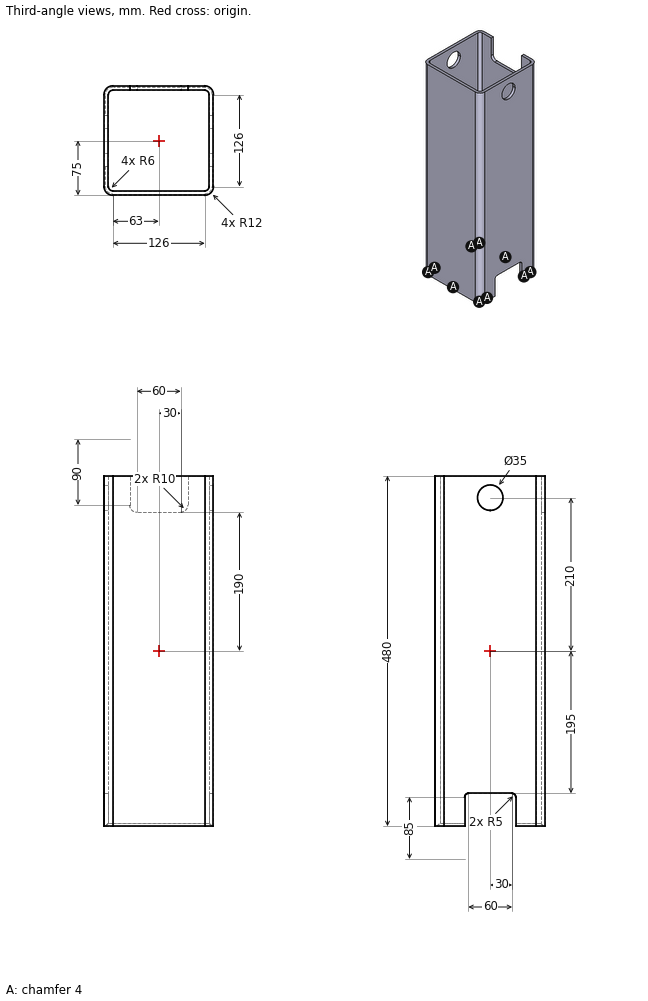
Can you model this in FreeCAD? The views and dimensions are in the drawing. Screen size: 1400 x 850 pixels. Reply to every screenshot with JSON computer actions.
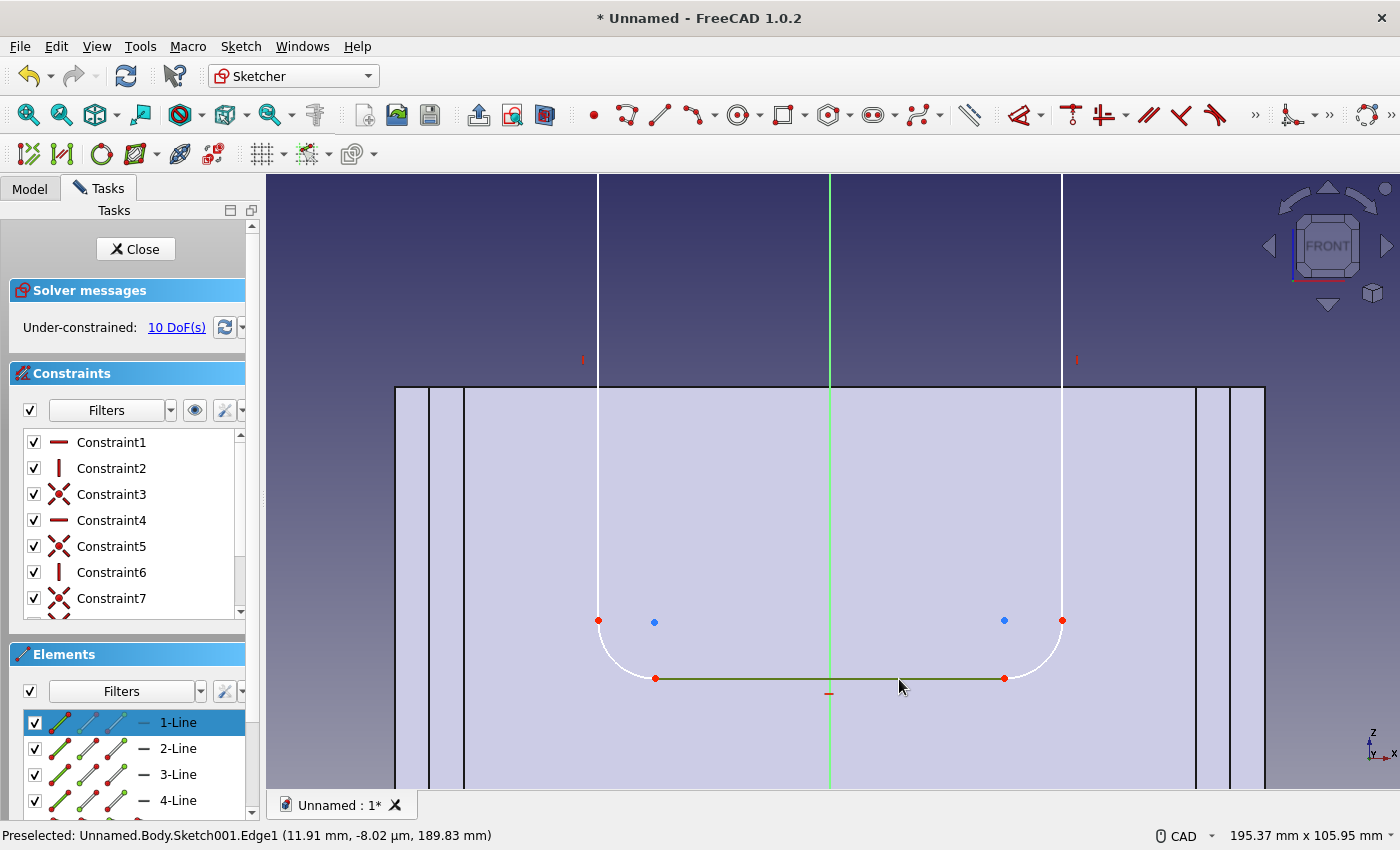
{"action": "left_click", "coordinate": [604, 647]}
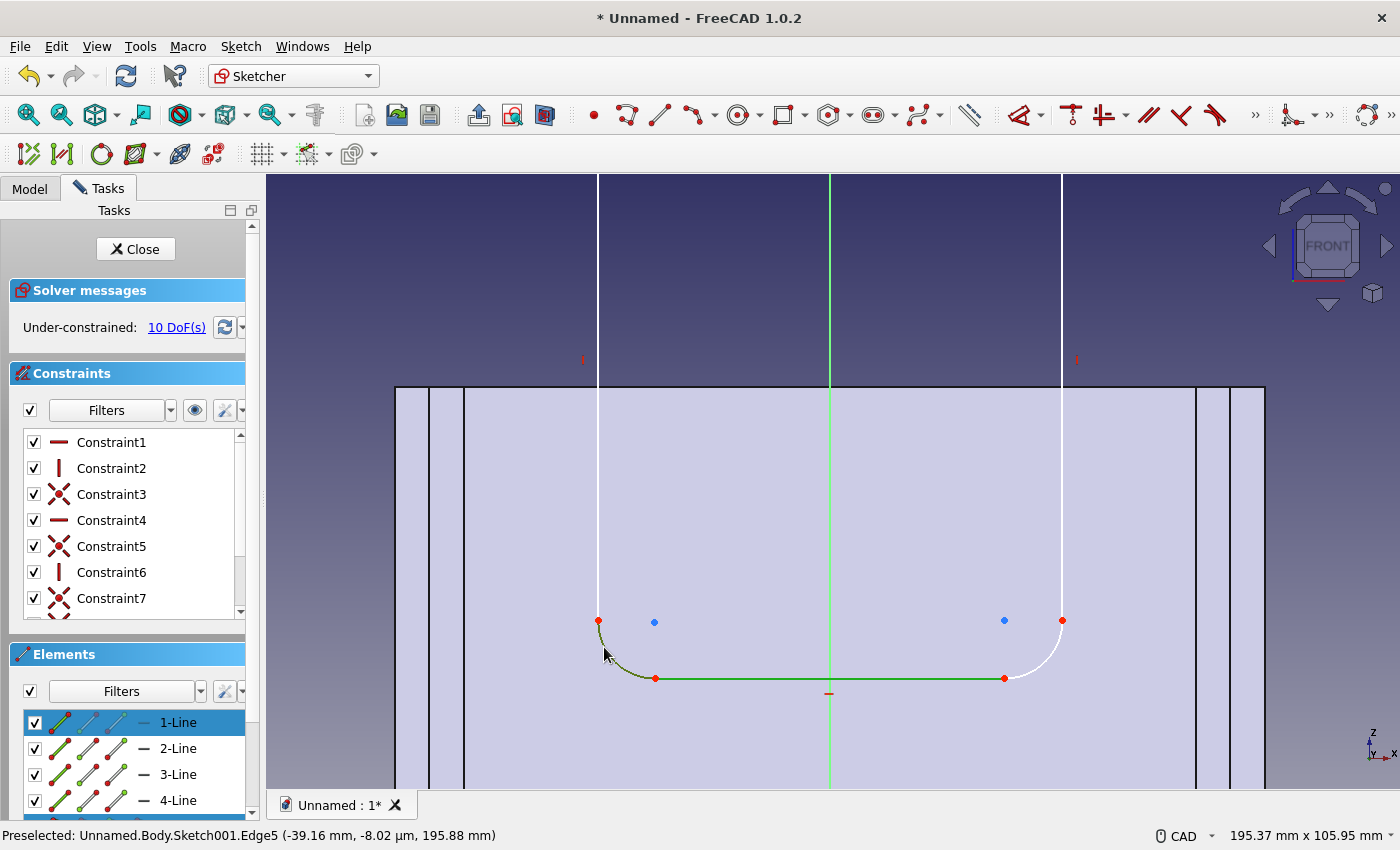
{"action": "key", "text": "t"}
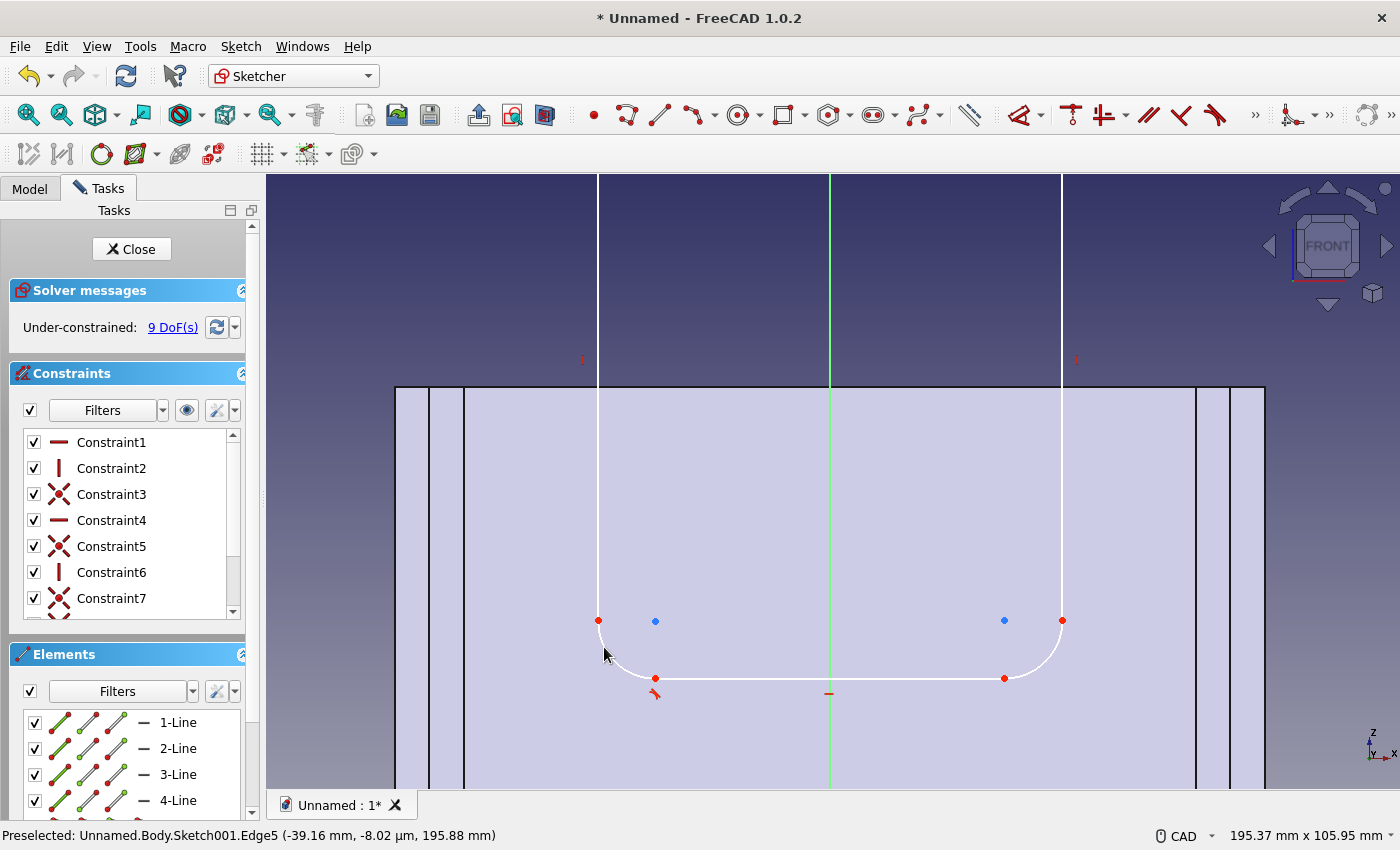
{"action": "left_click", "coordinate": [899, 679]}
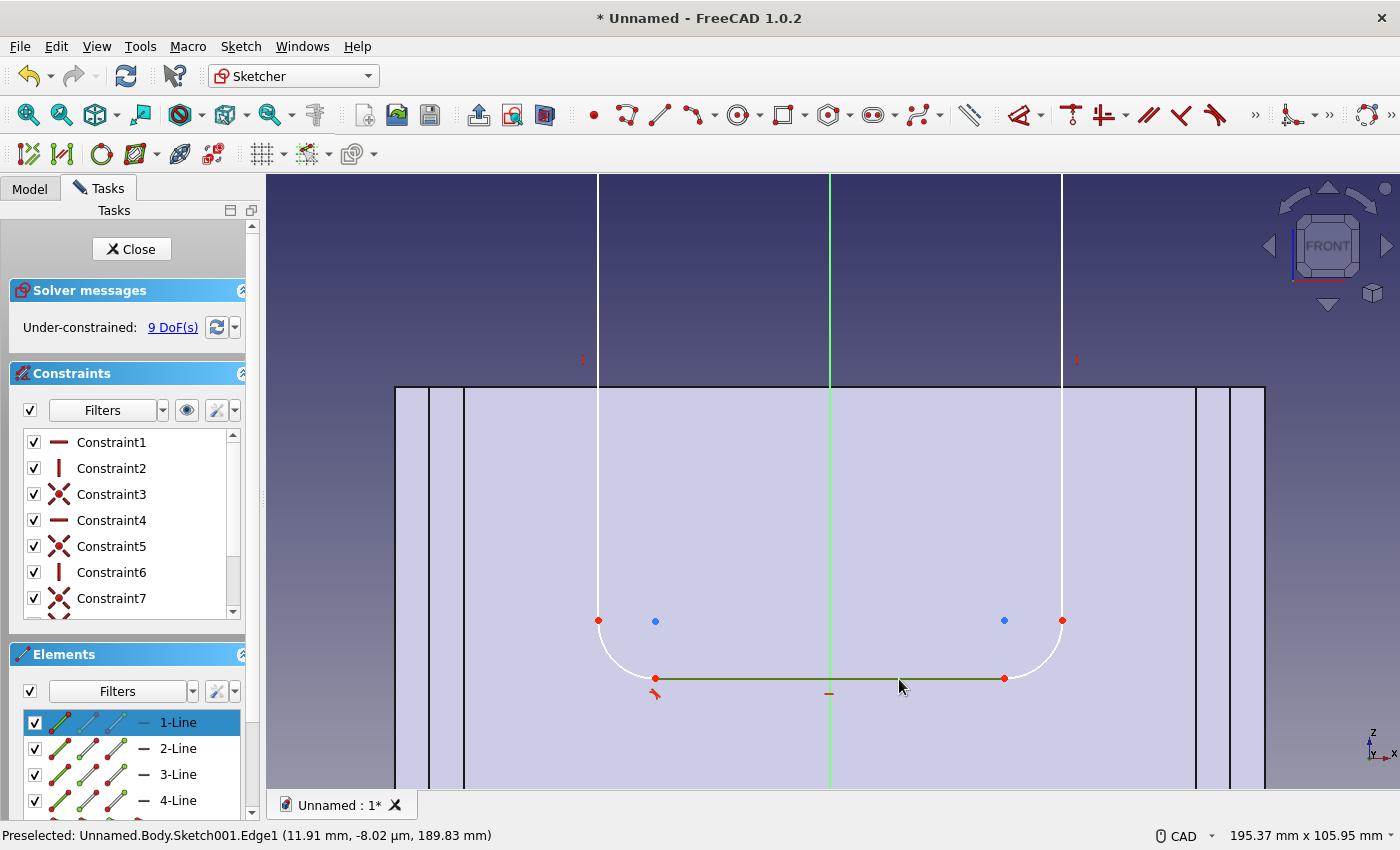
{"action": "left_click", "coordinate": [1031, 672]}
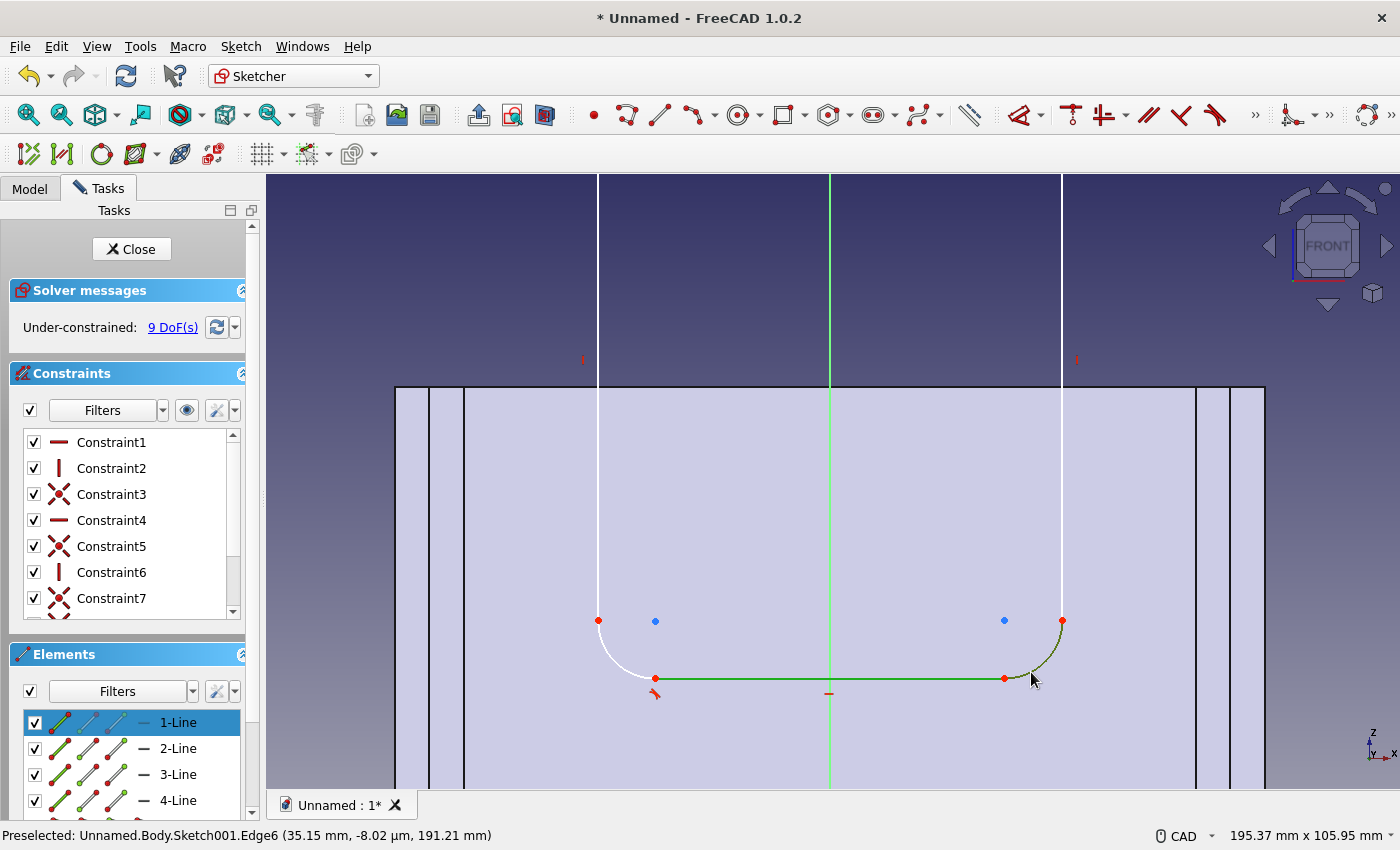
{"action": "key", "text": "t"}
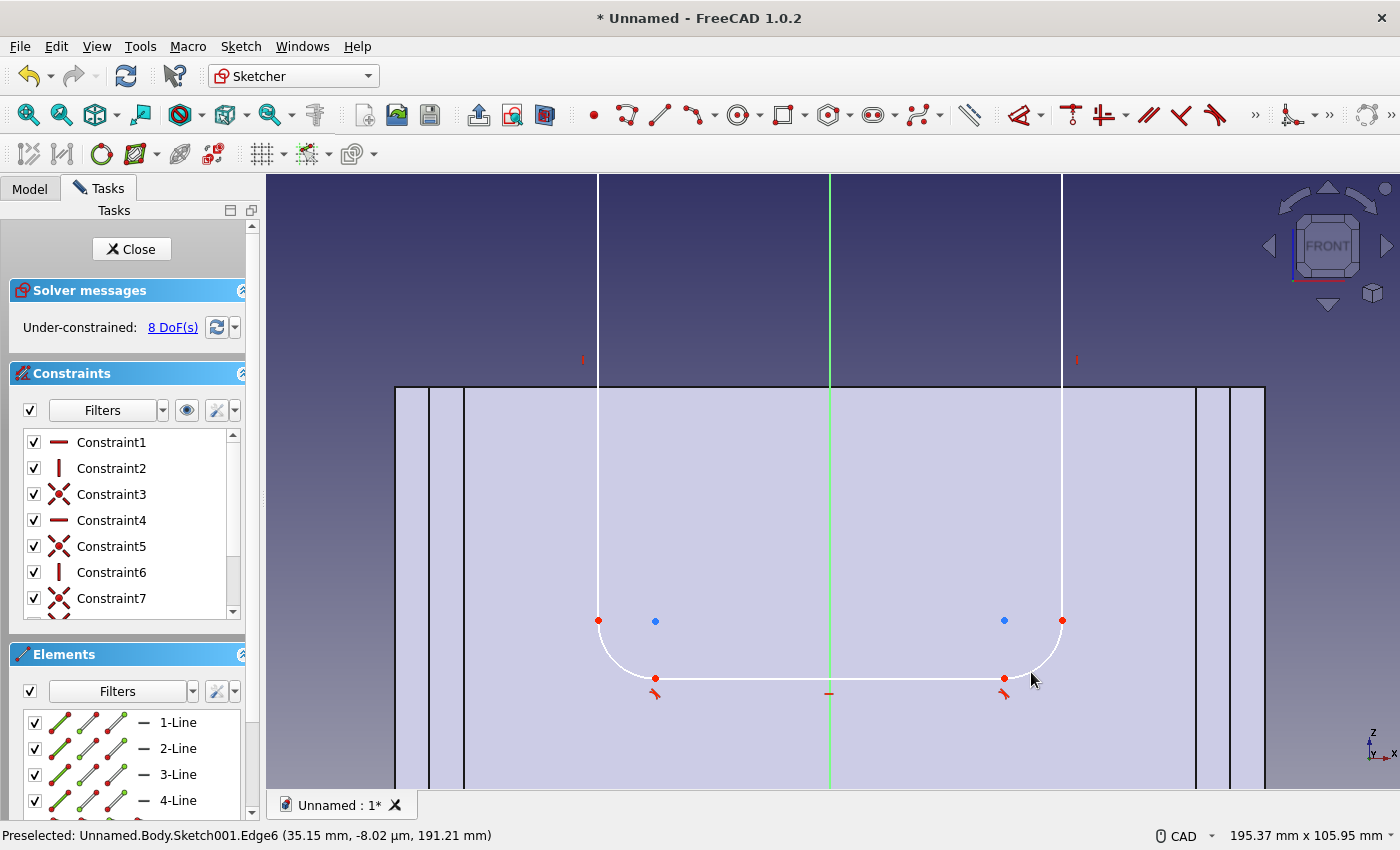
{"action": "left_click", "coordinate": [598, 464]}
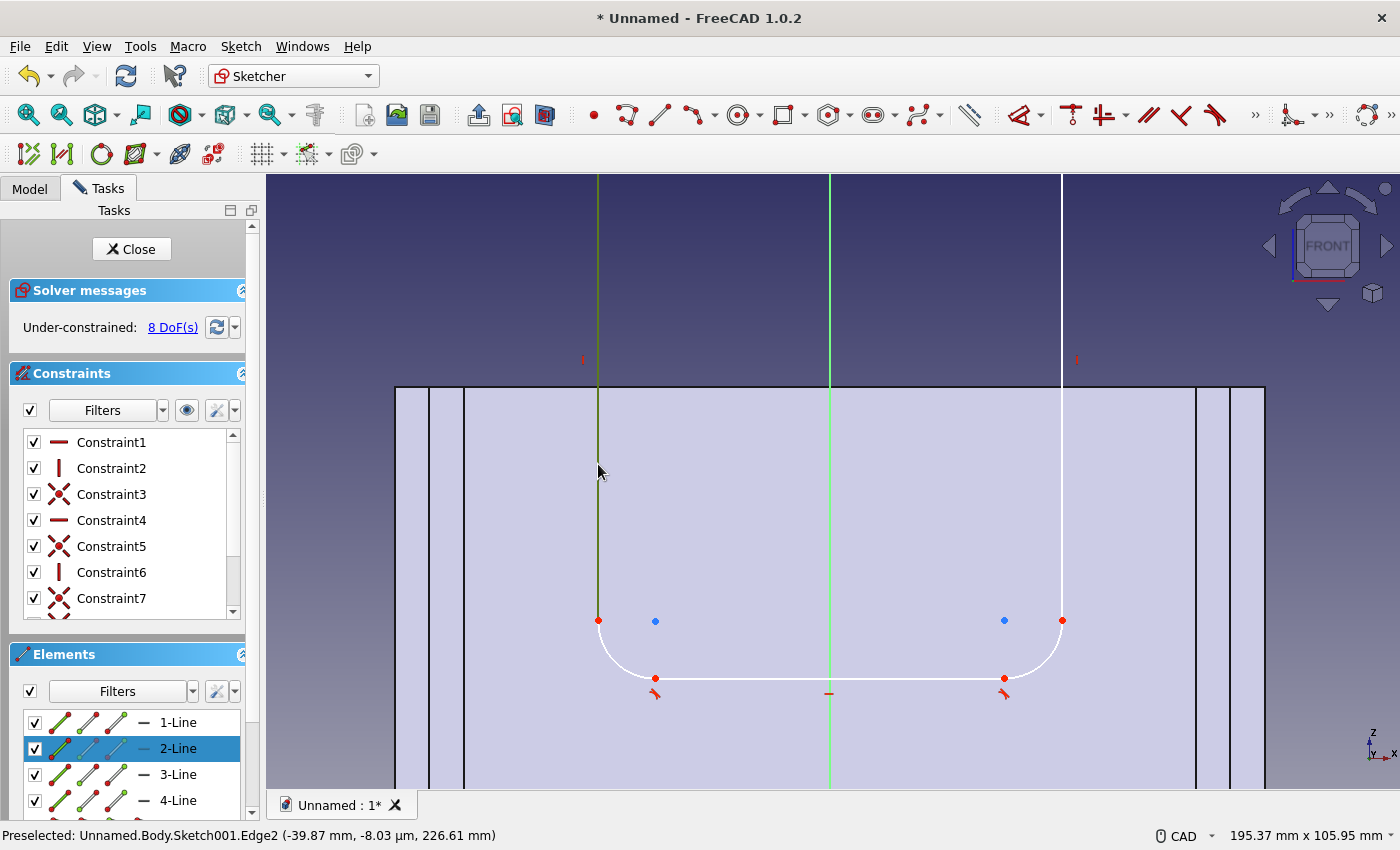
{"action": "left_click", "coordinate": [604, 647]}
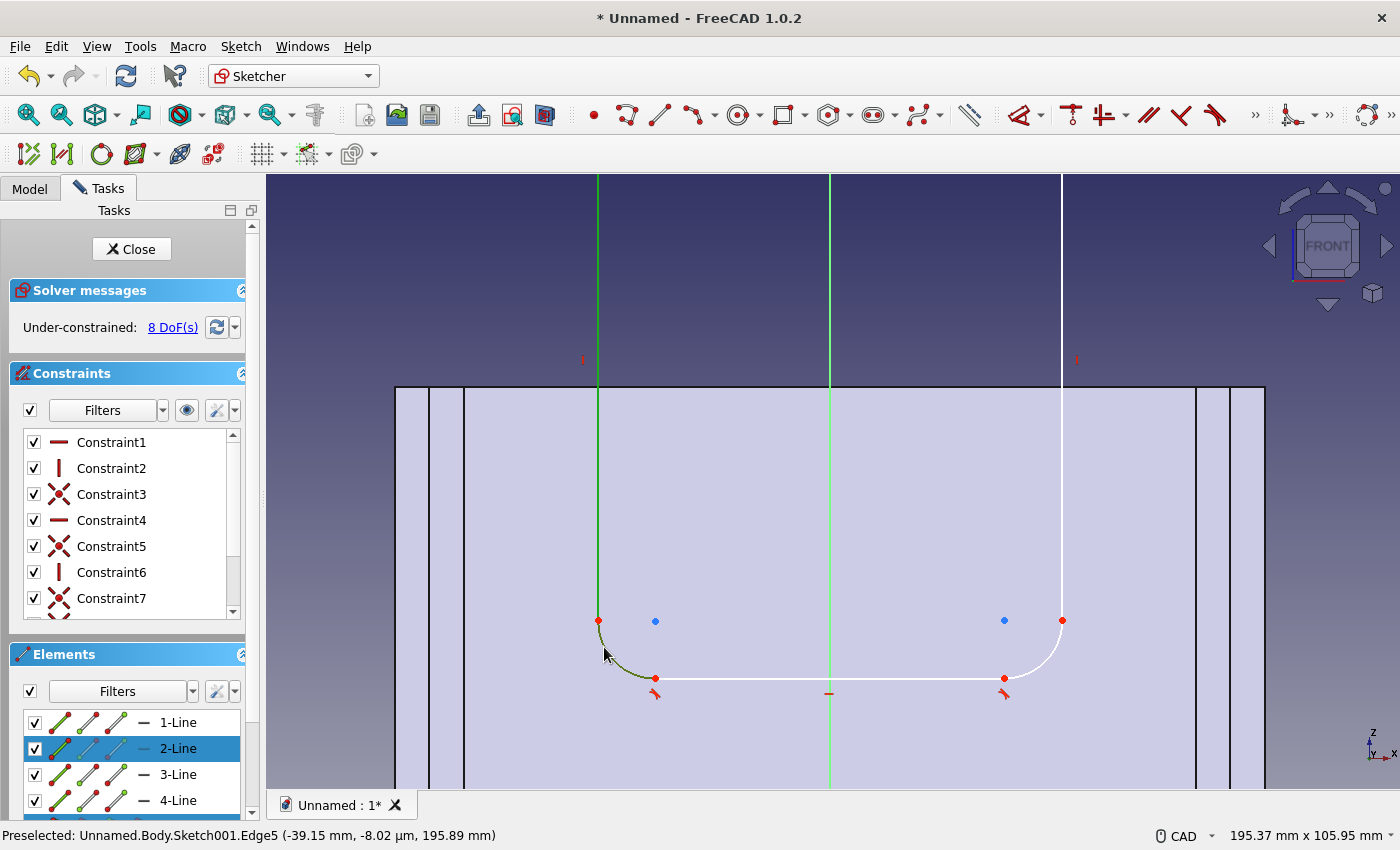
{"action": "left_click", "coordinate": [1215, 116]}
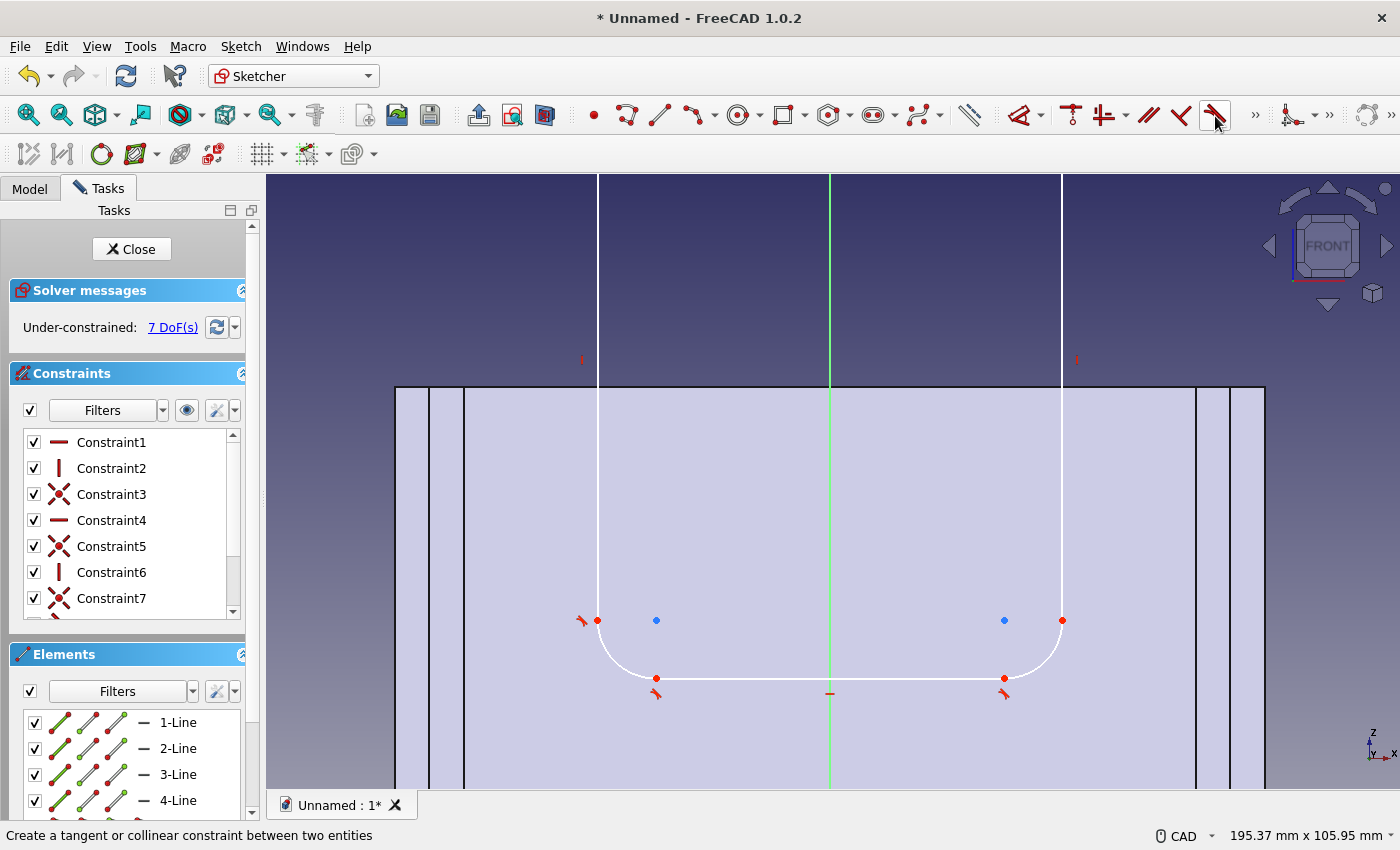
{"action": "left_click", "coordinate": [1062, 255]}